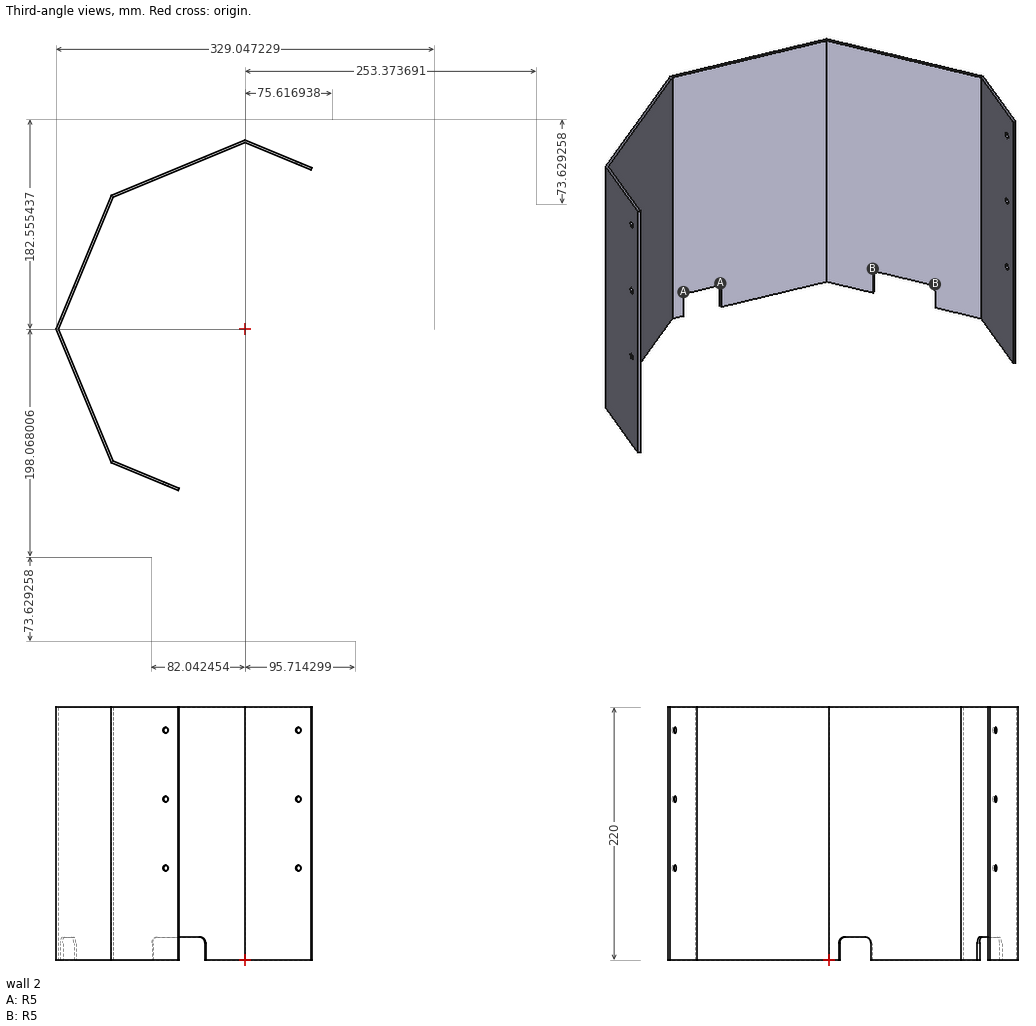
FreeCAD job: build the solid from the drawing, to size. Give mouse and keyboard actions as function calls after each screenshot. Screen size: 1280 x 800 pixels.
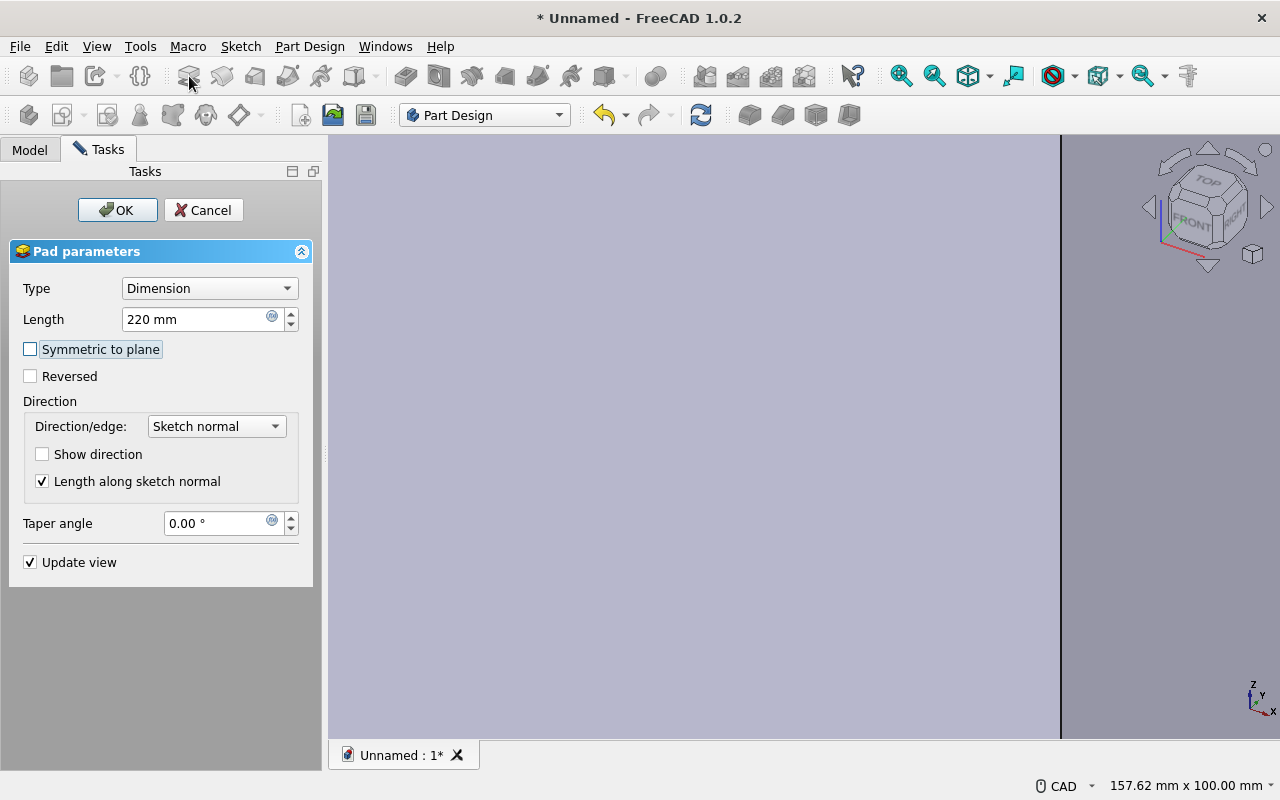
click(118, 210)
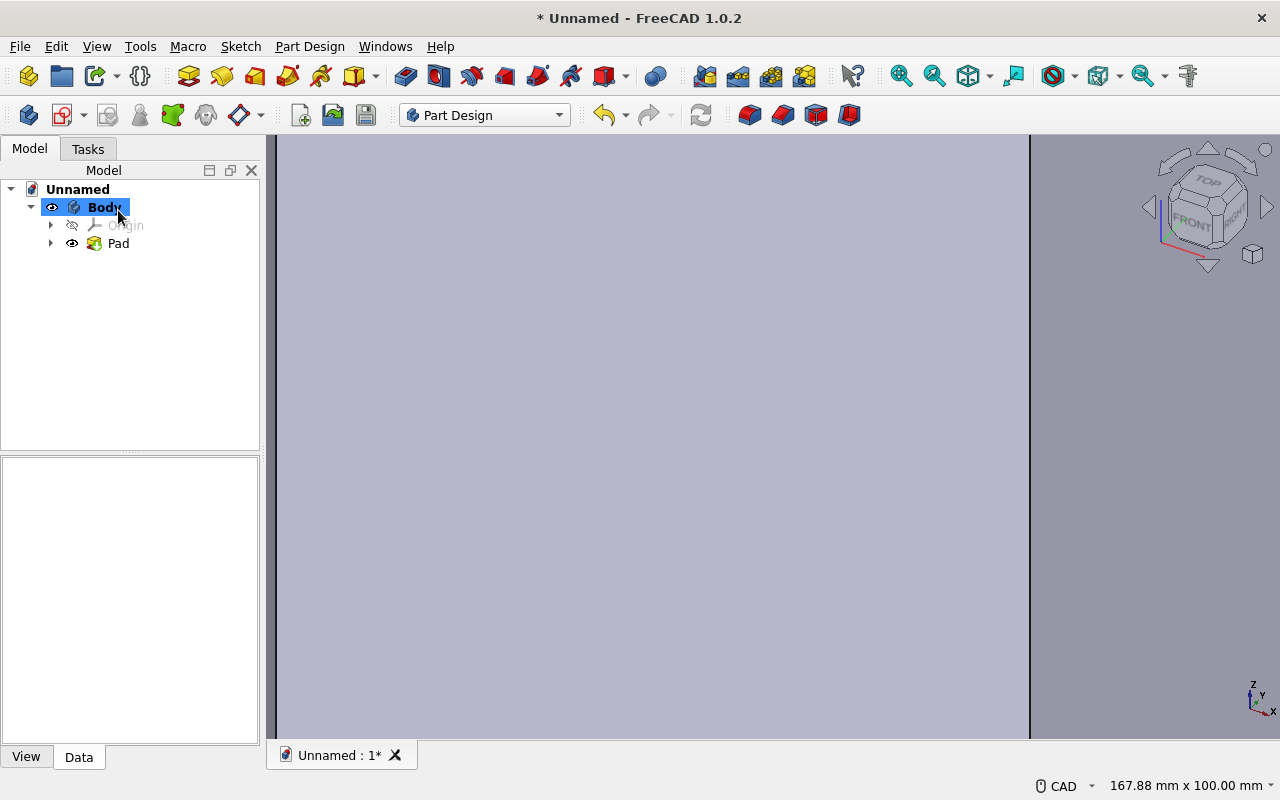
click(902, 76)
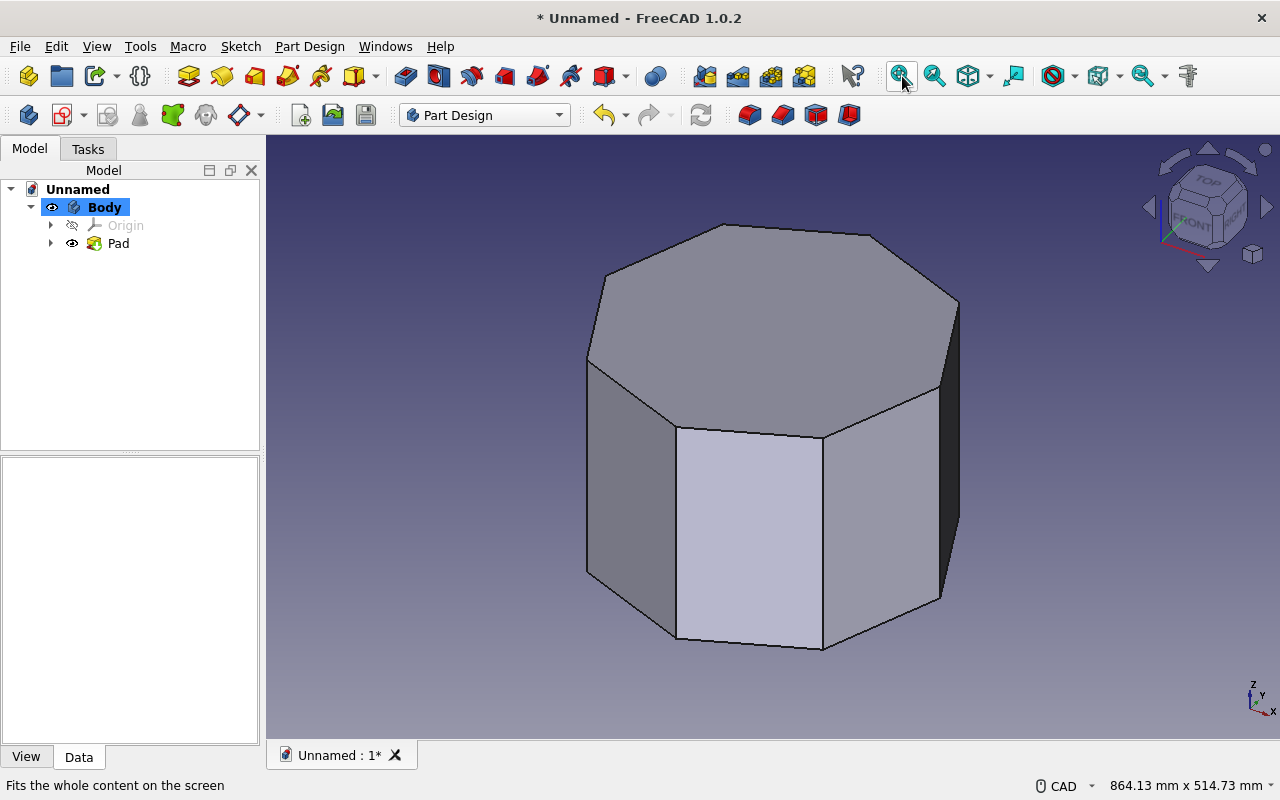
click(773, 330)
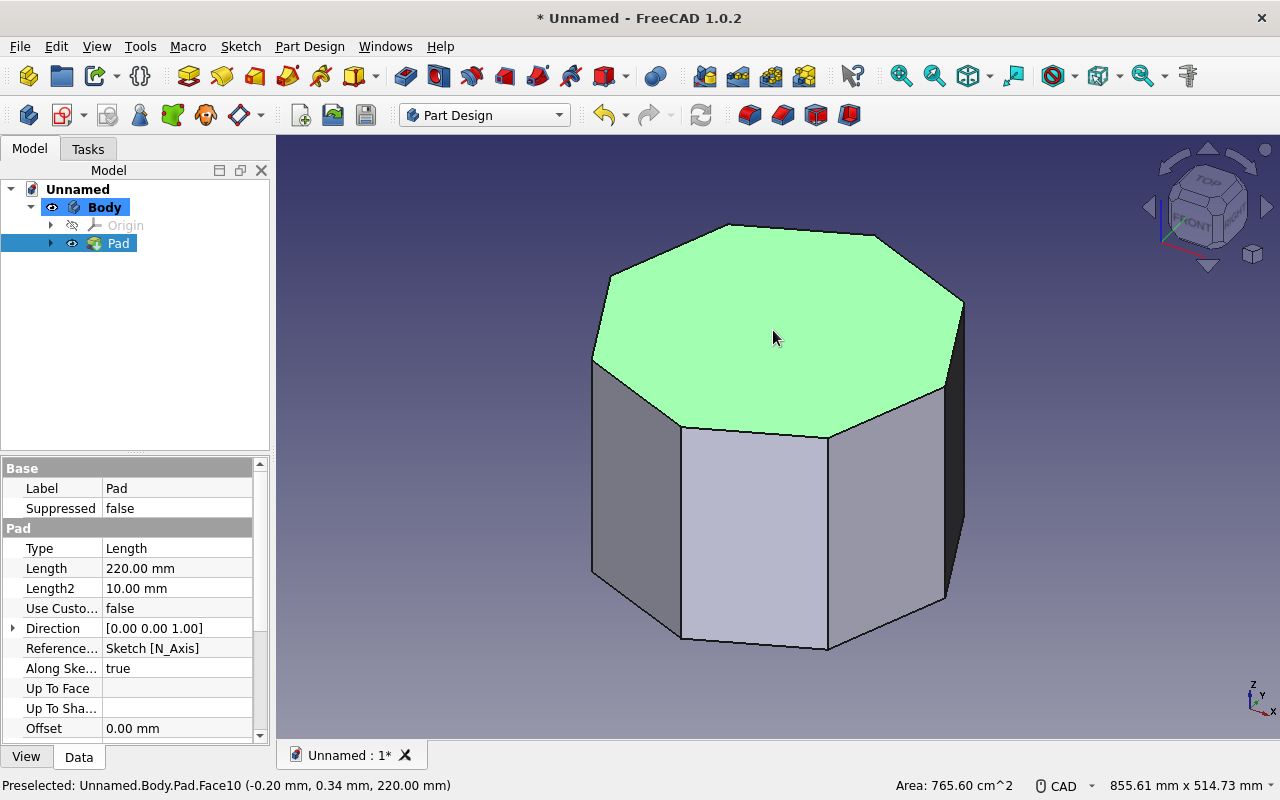
key(0)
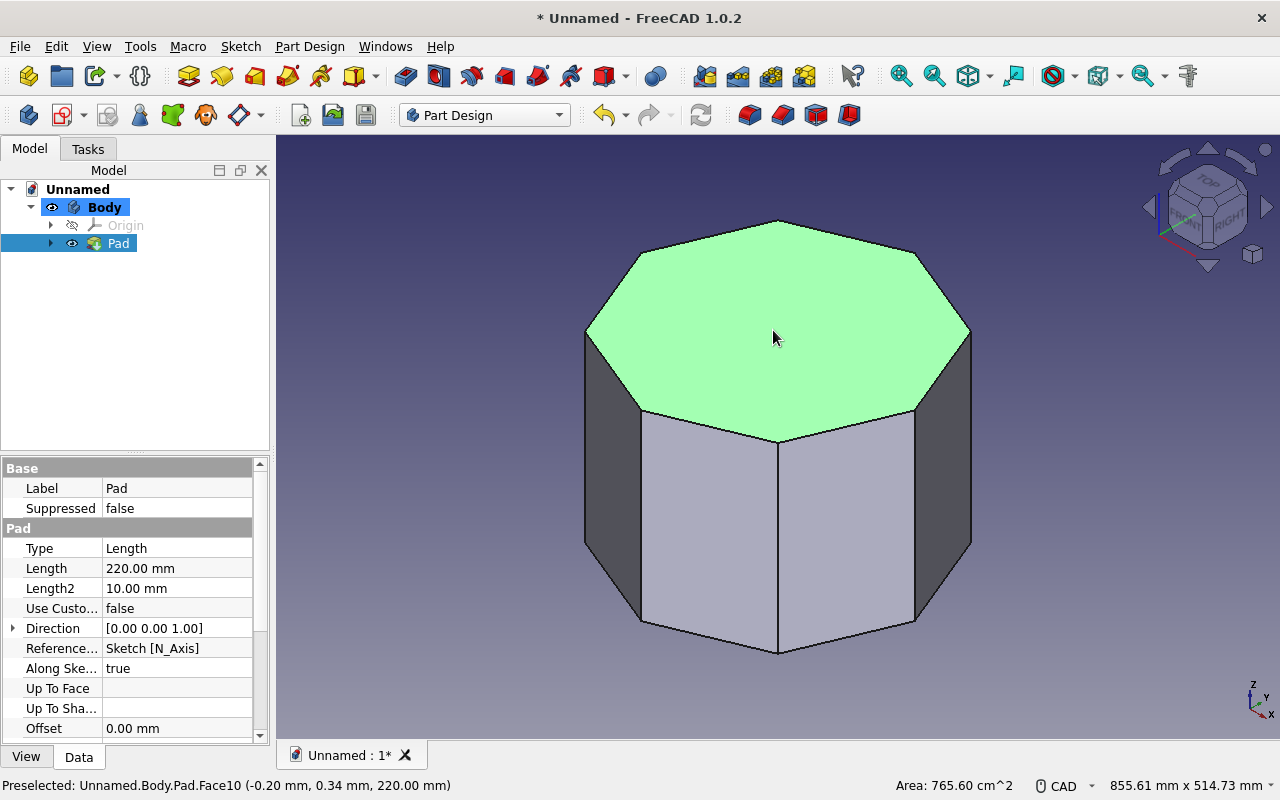
key(2)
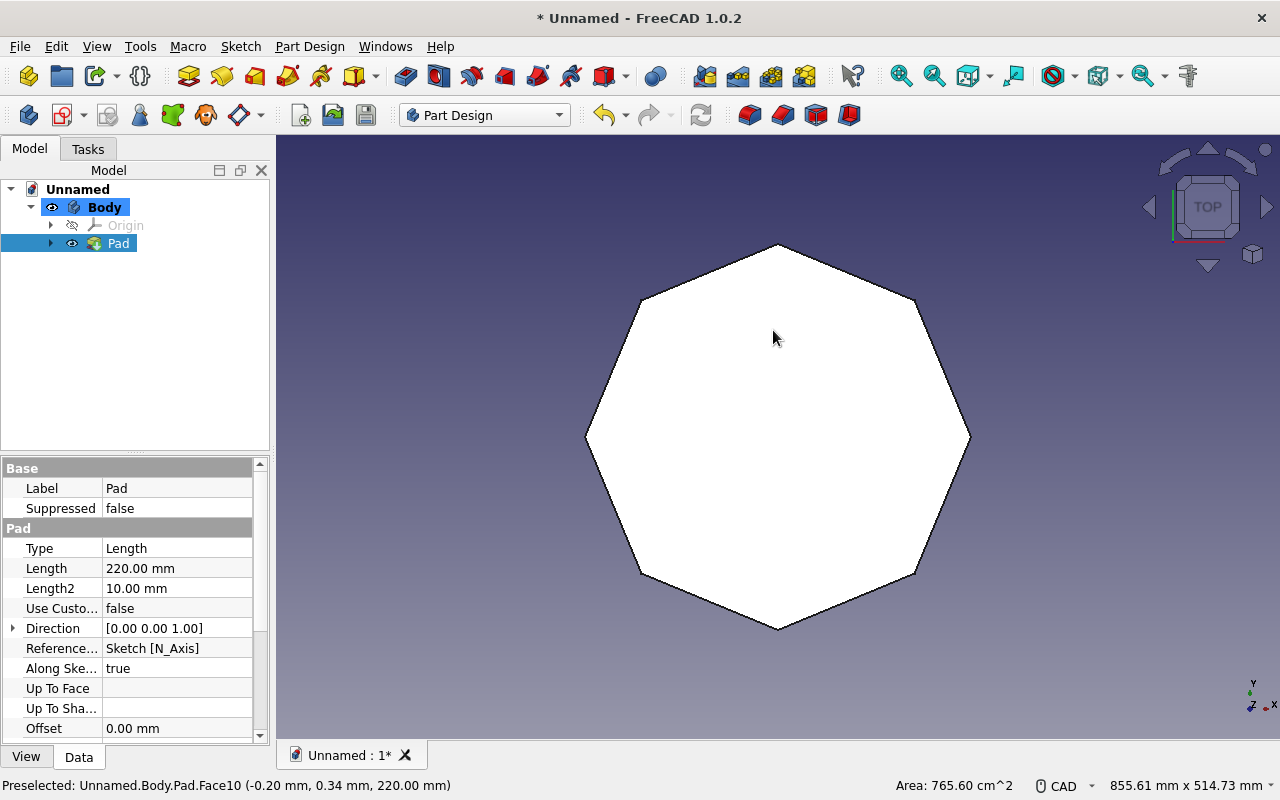
key(1)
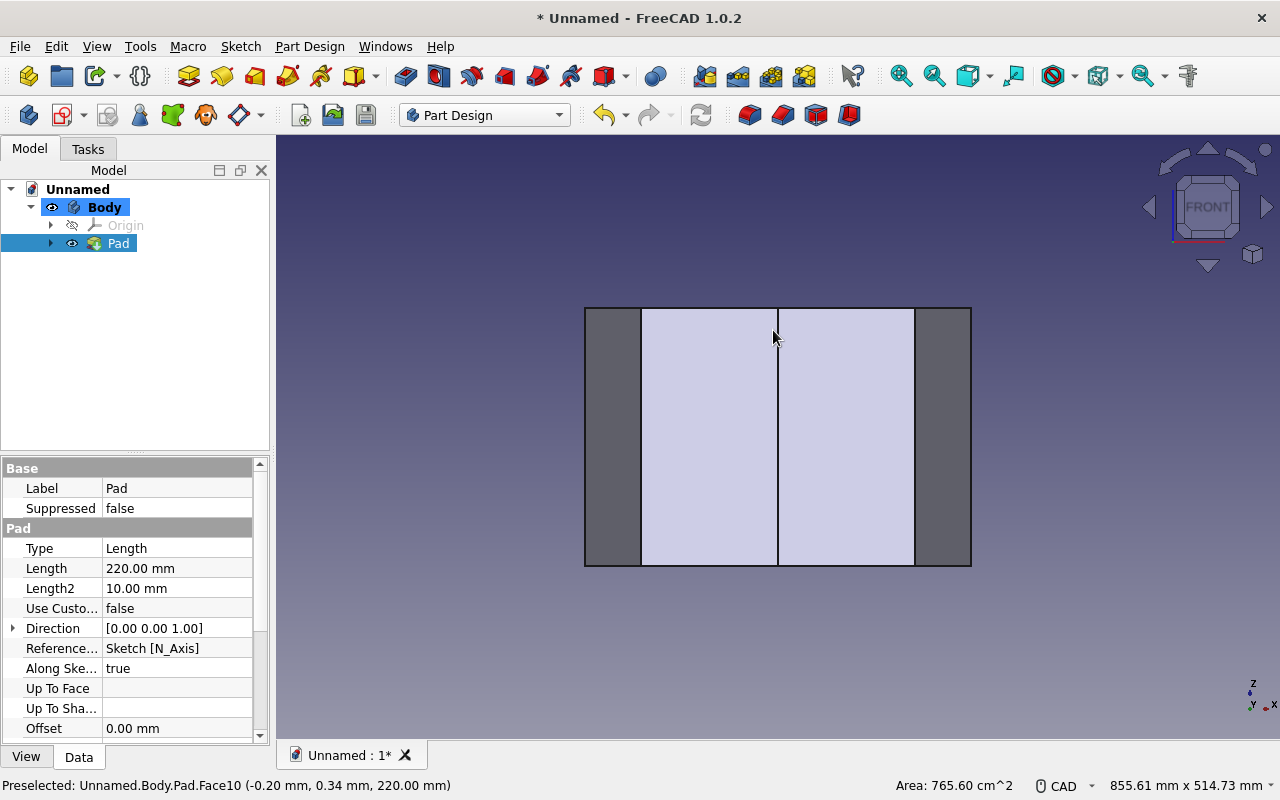
click(902, 76)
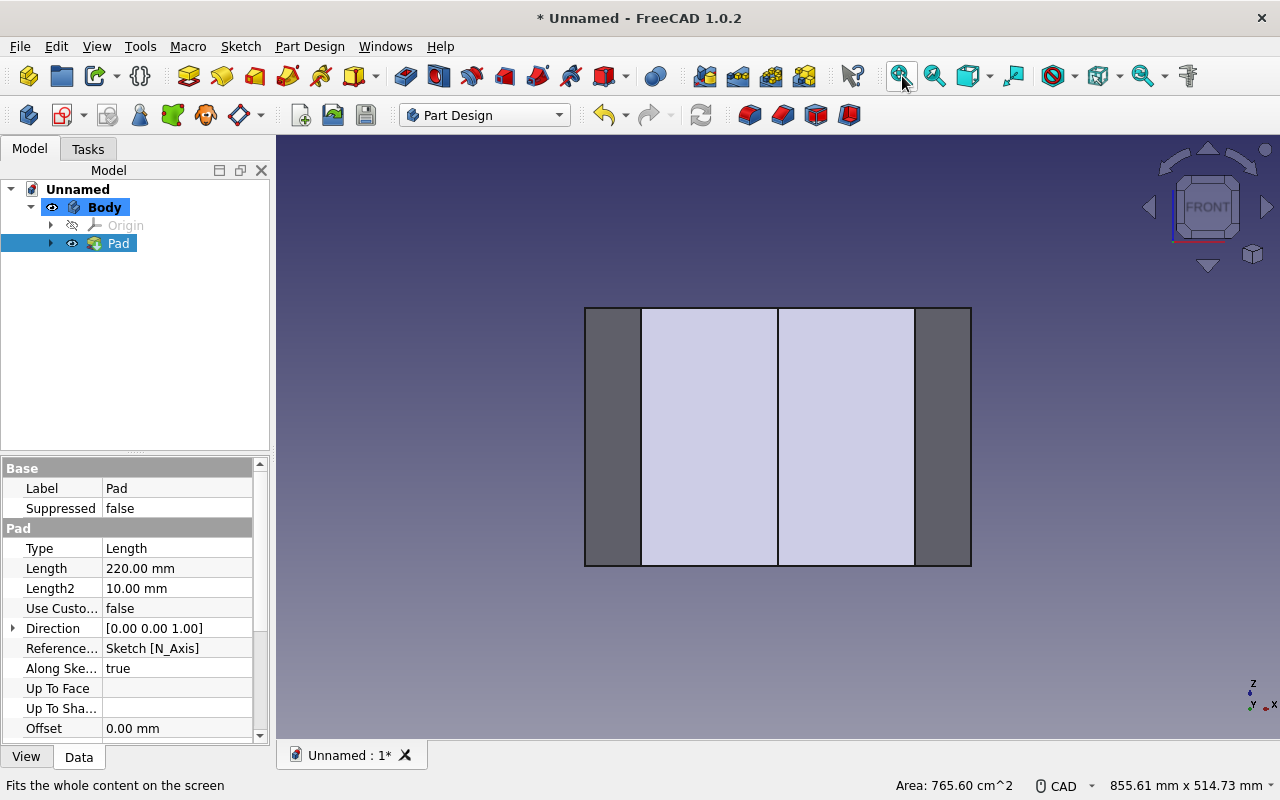
key(3)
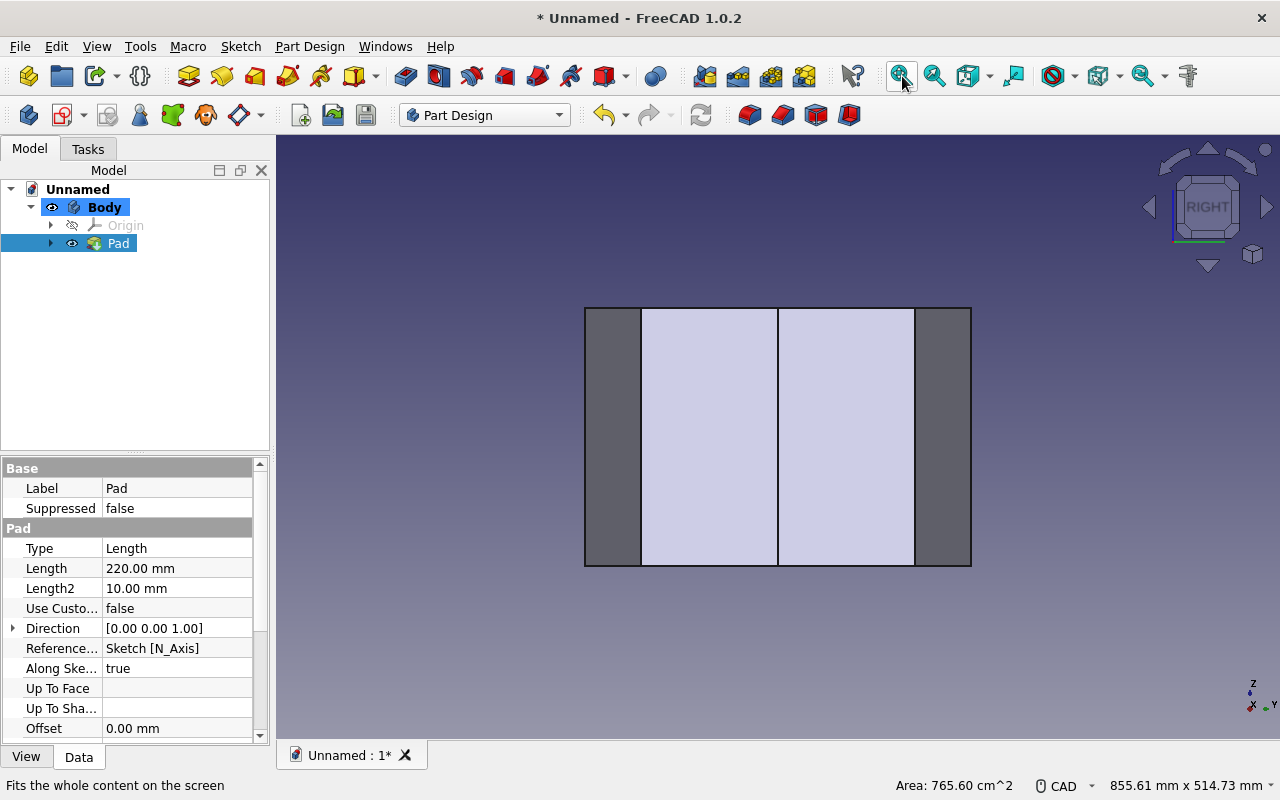
click(902, 76)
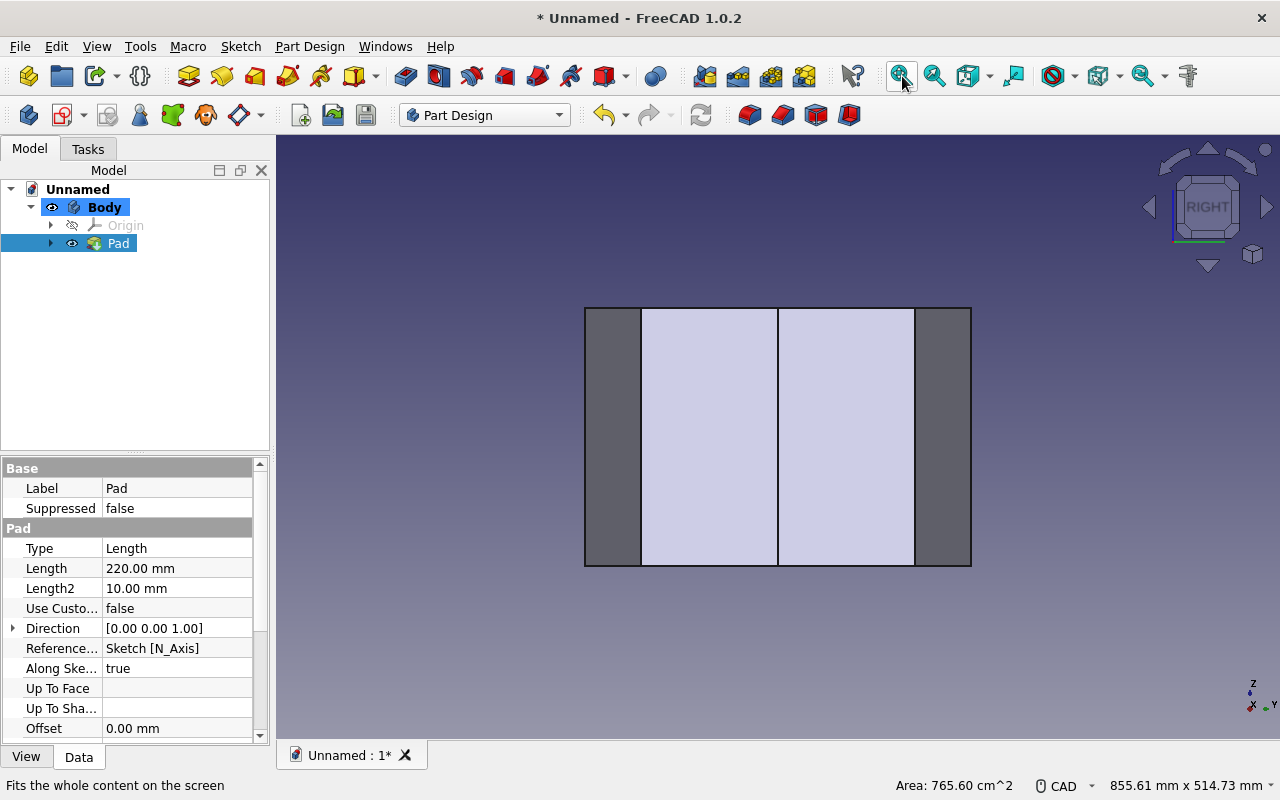
key(5)